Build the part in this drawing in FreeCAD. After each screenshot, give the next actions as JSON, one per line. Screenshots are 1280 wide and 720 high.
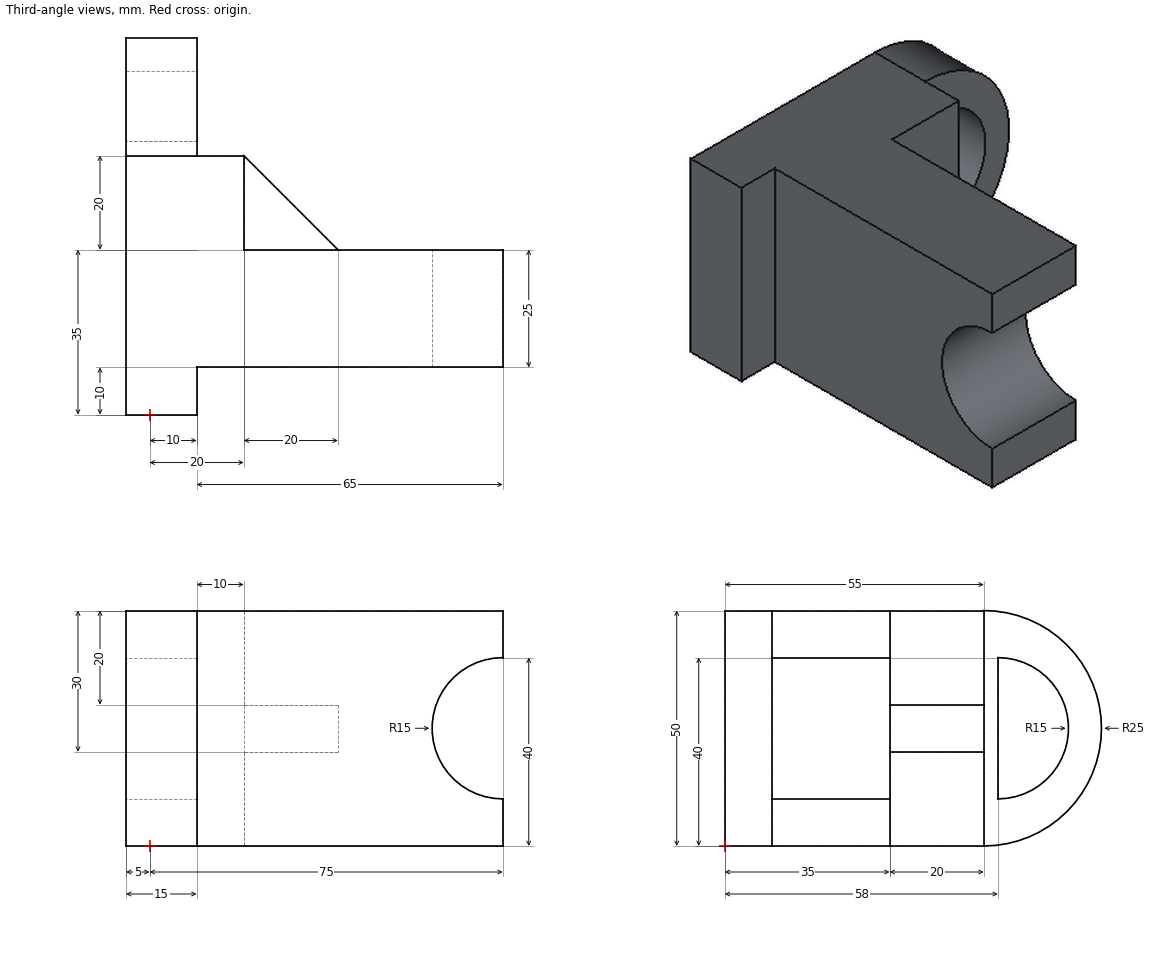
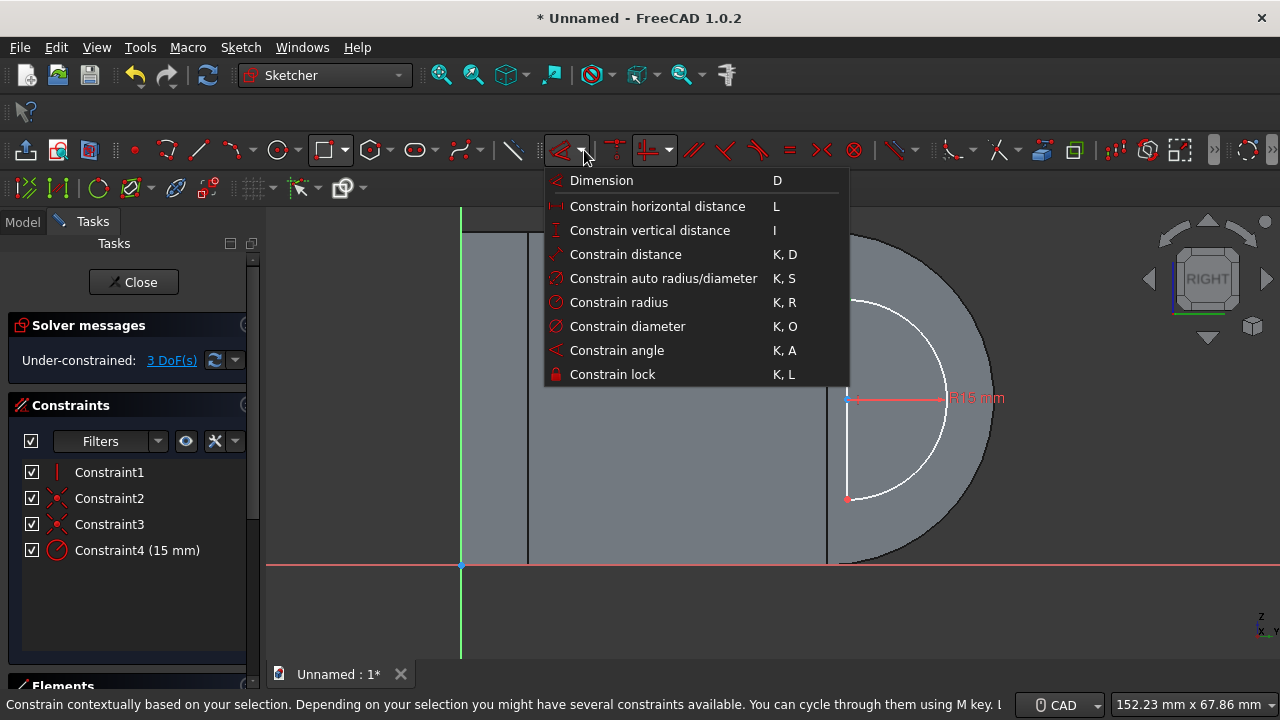
{"action": "left_click", "coordinate": [697, 206]}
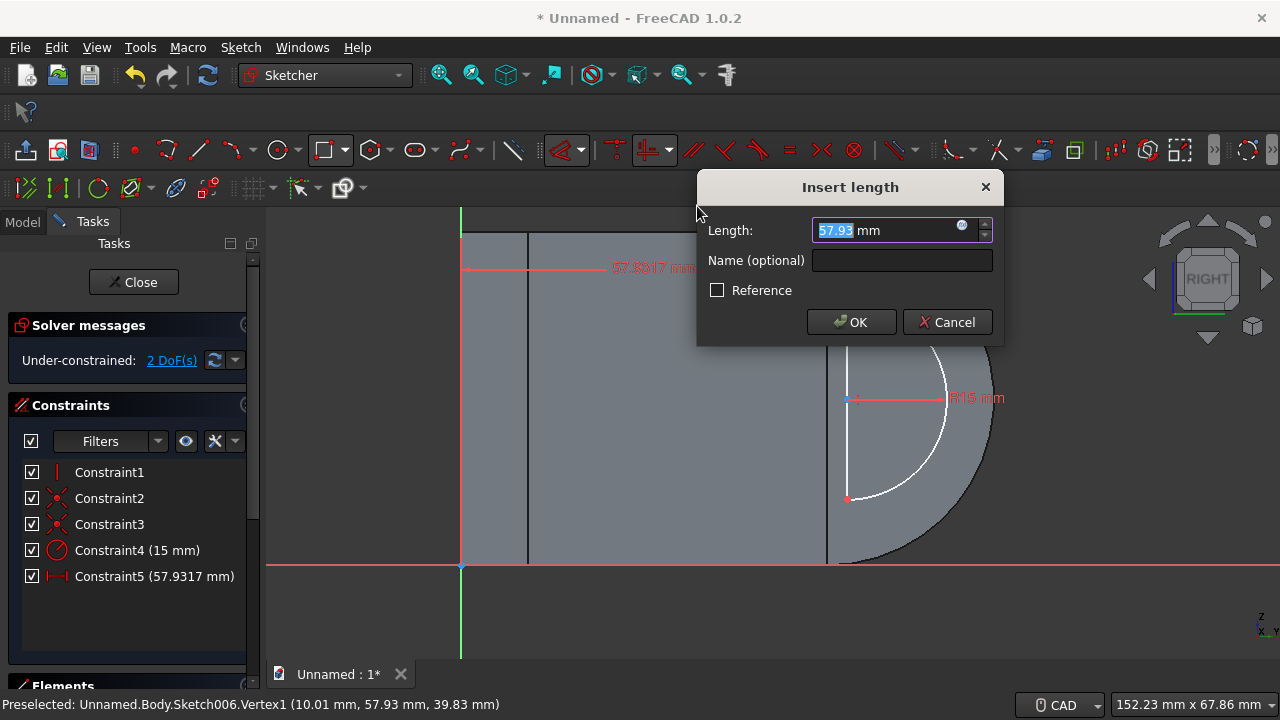
{"action": "type", "text": "58"}
{"action": "key", "text": "Return"}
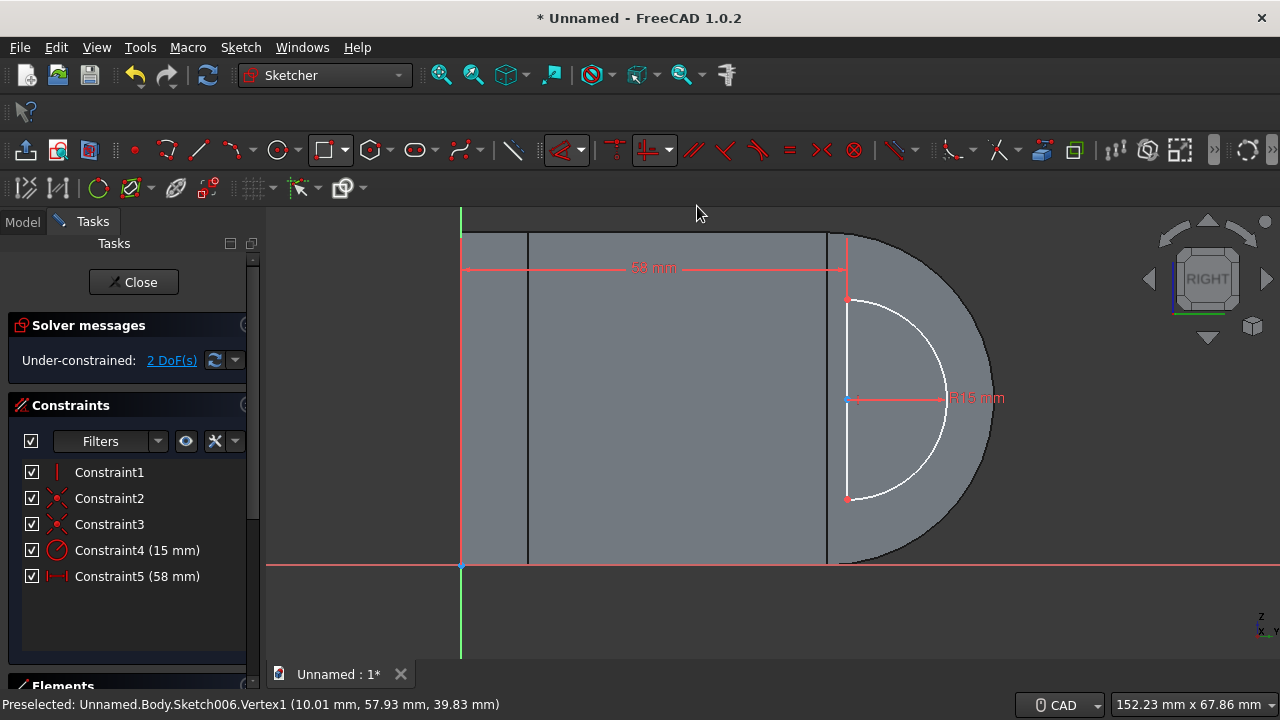
{"action": "left_click", "coordinate": [847, 300]}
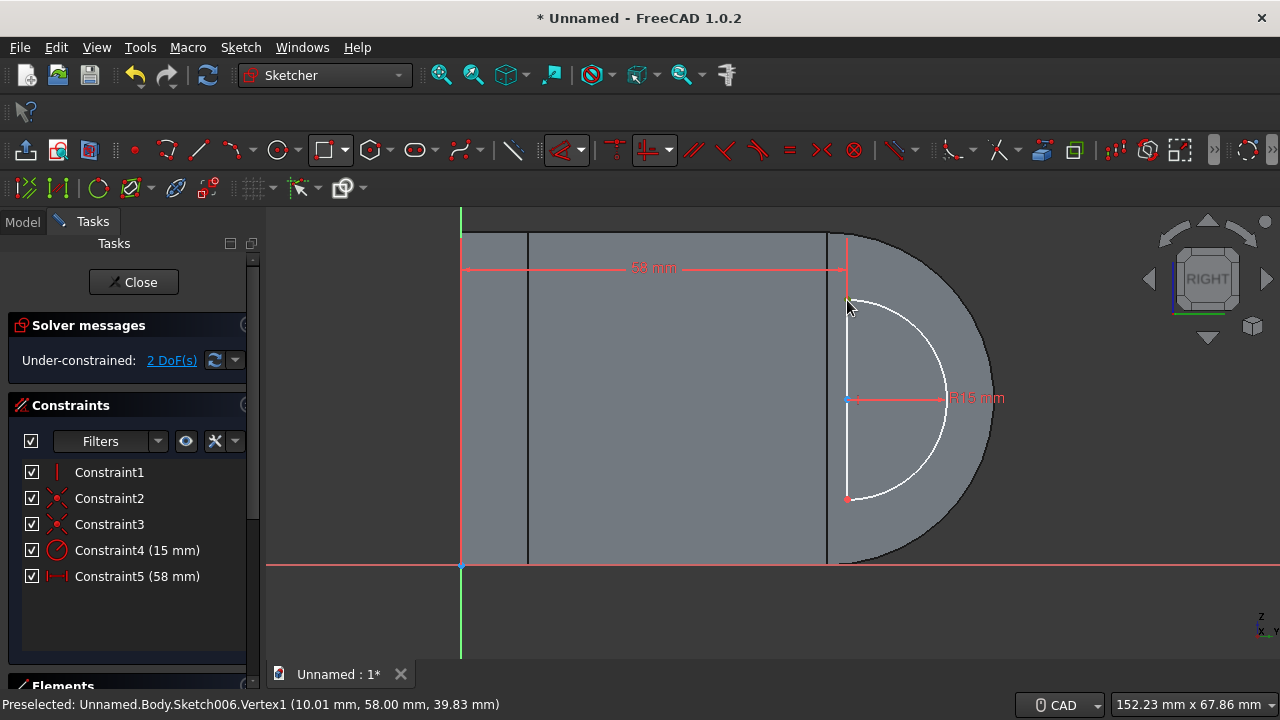
{"action": "key", "text": "i"}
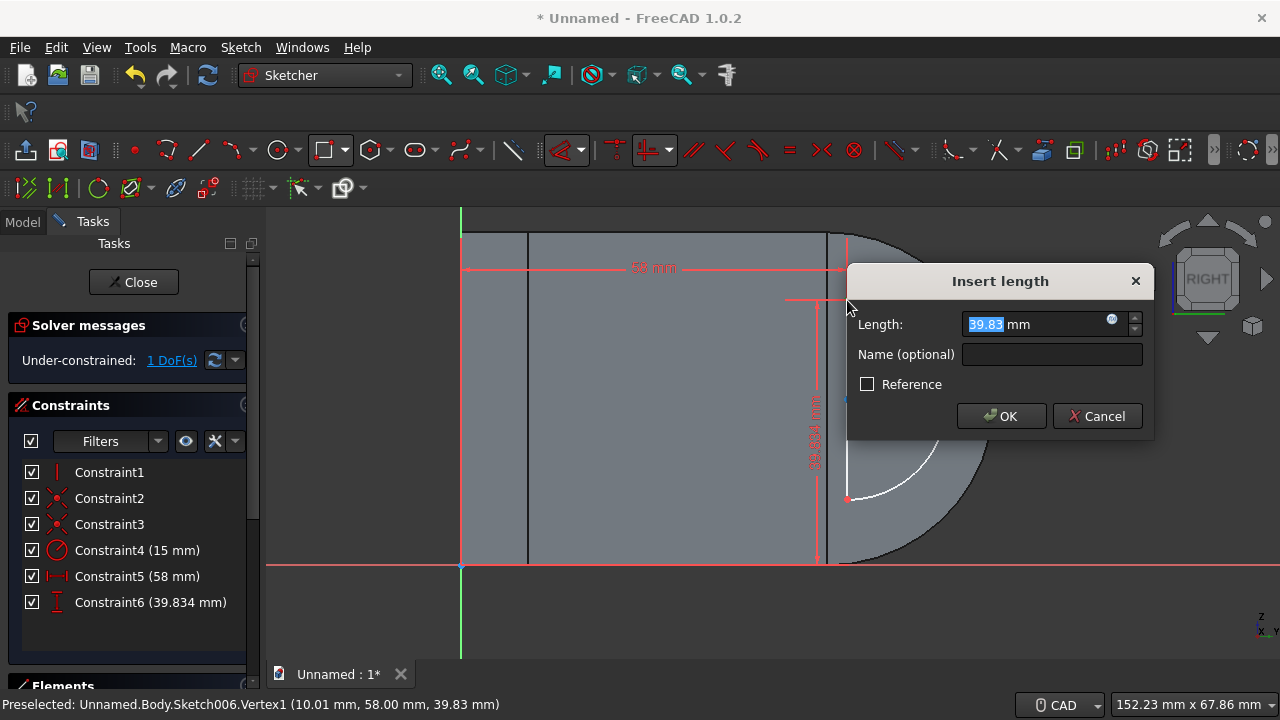
{"action": "type", "text": "40"}
{"action": "key", "text": "Return"}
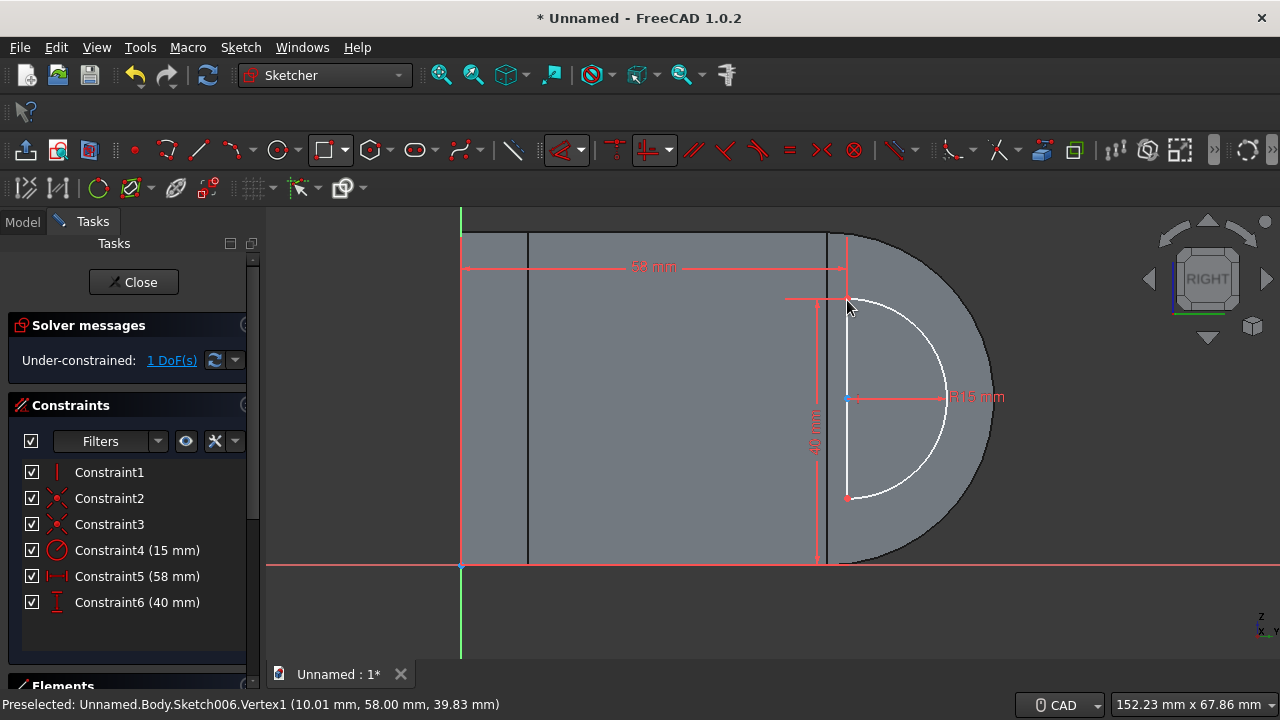
{"action": "left_click", "coordinate": [847, 399]}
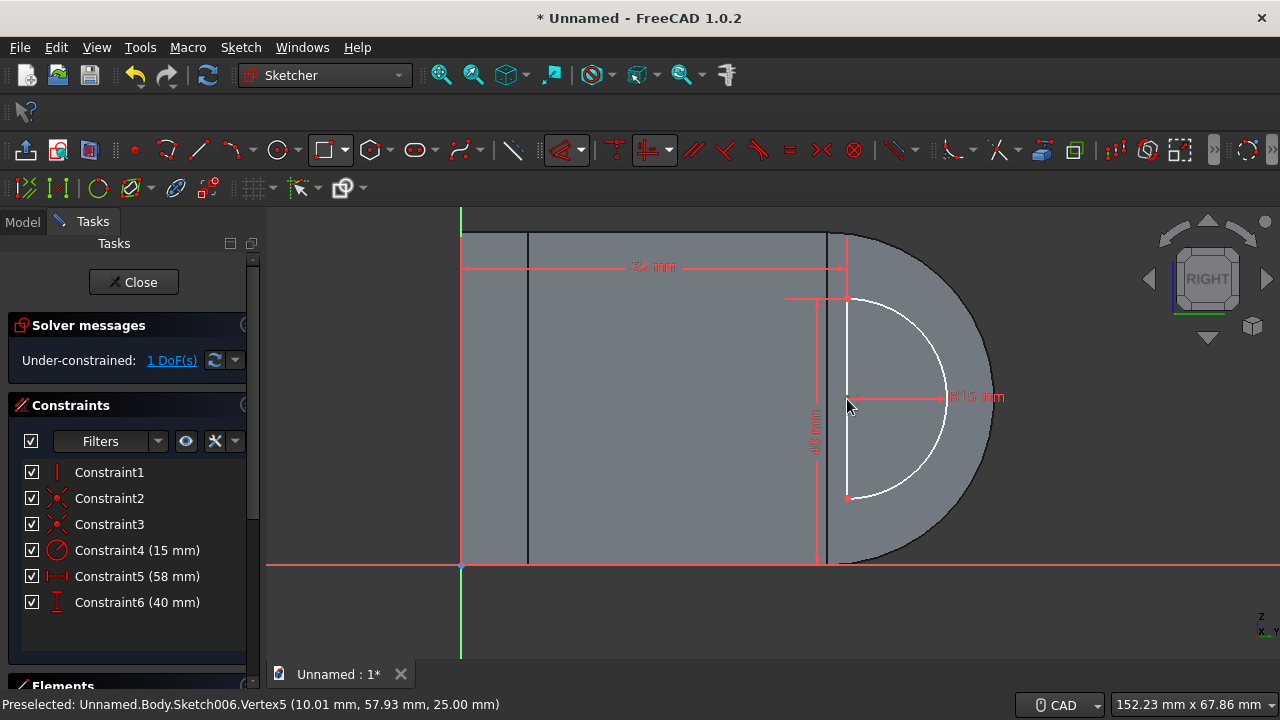
{"action": "left_click", "coordinate": [584, 150]}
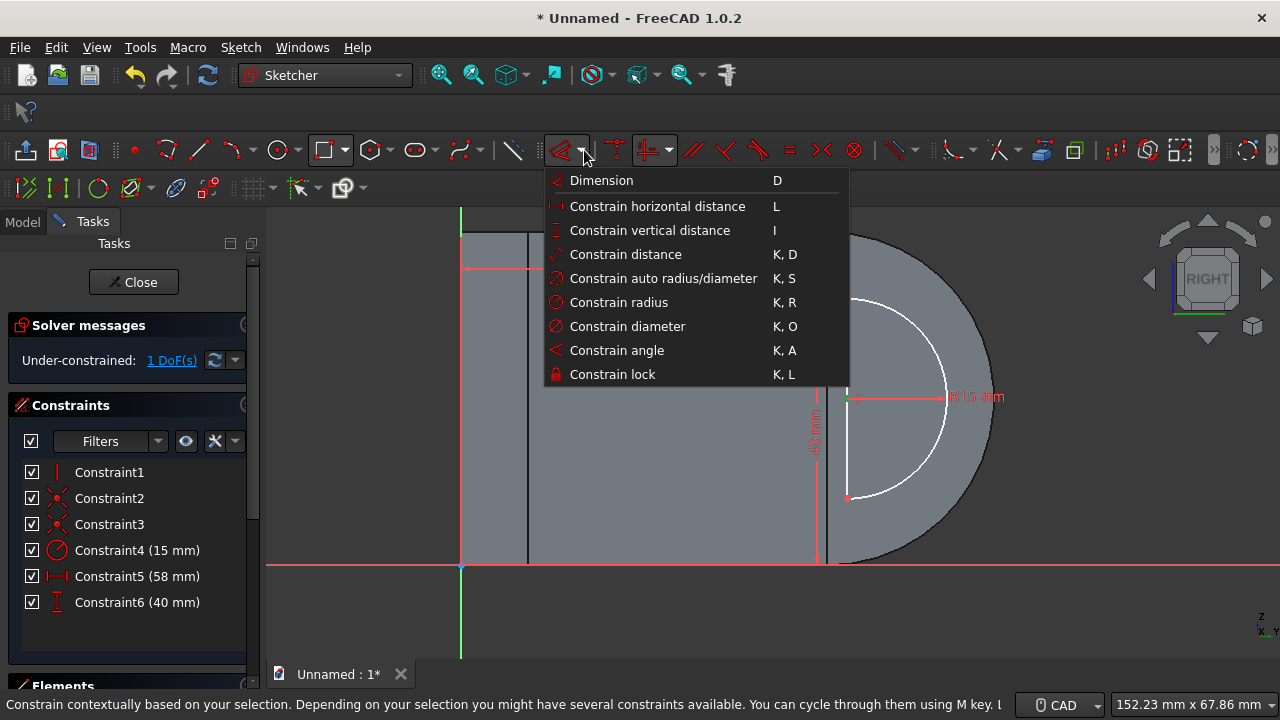
{"action": "left_click", "coordinate": [697, 206]}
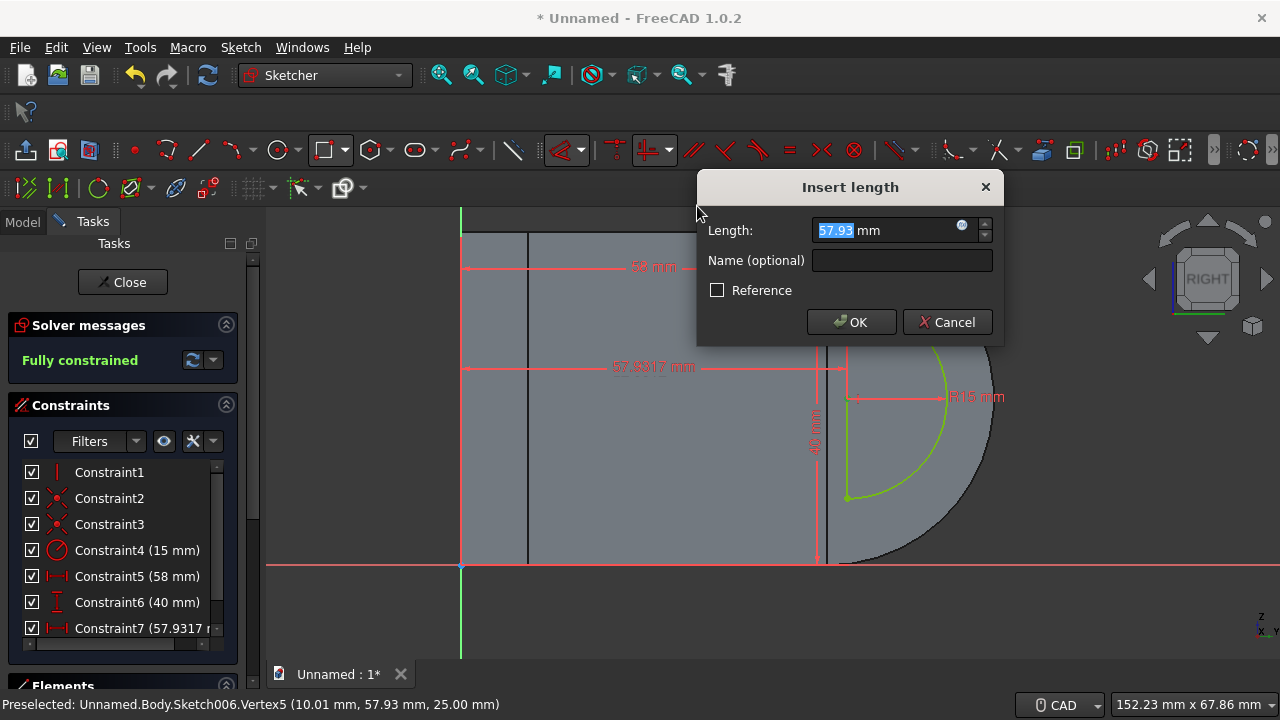
{"action": "type", "text": "58"}
{"action": "key", "text": "Return"}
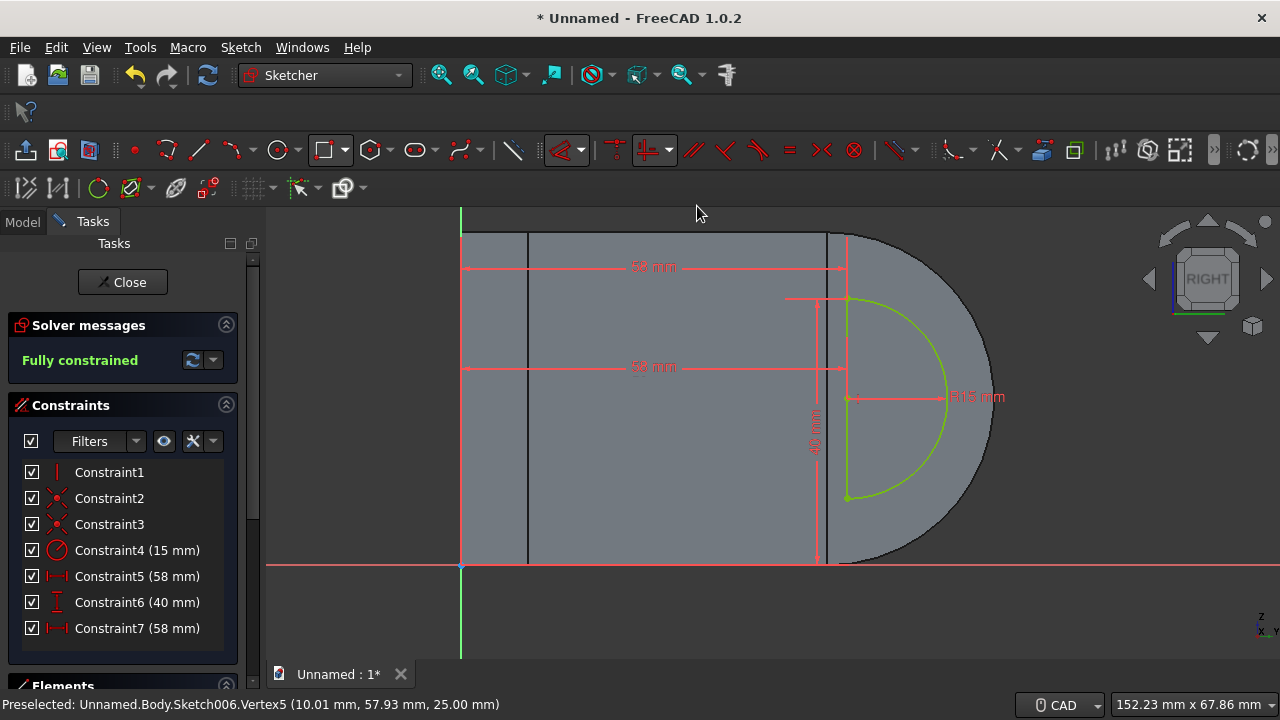
{"action": "left_click", "coordinate": [123, 282]}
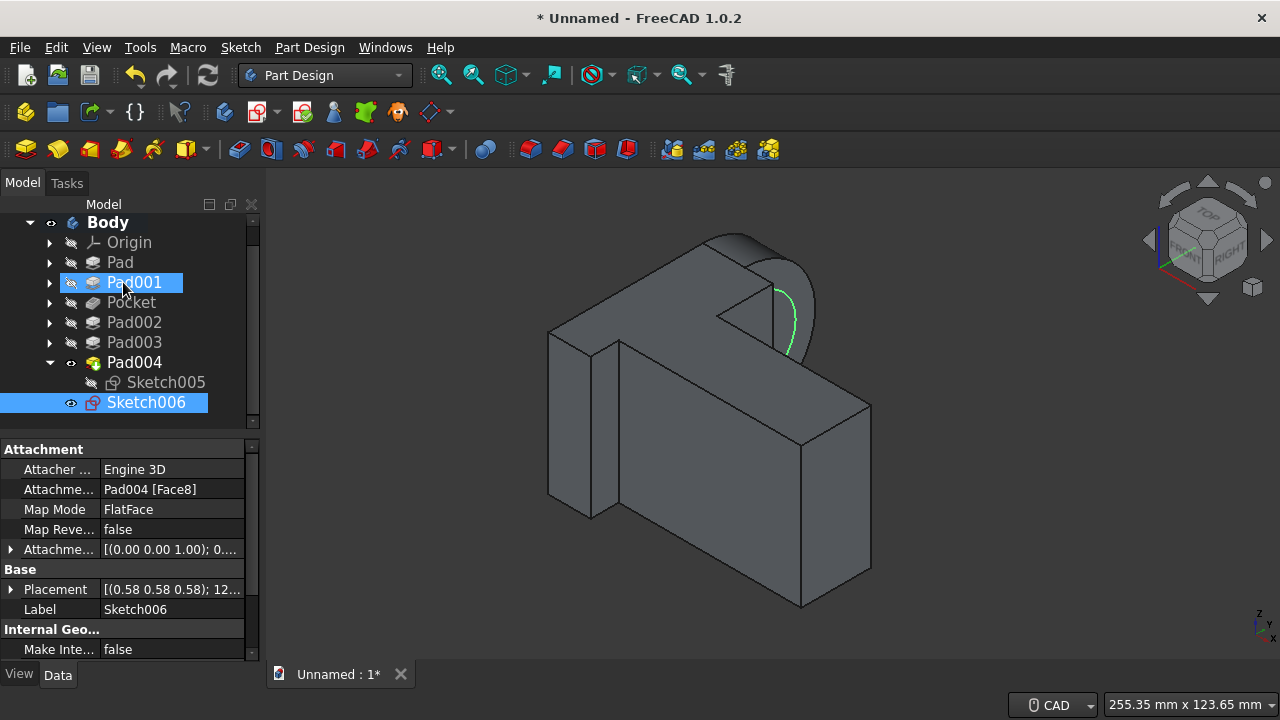
{"action": "left_click", "coordinate": [240, 150]}